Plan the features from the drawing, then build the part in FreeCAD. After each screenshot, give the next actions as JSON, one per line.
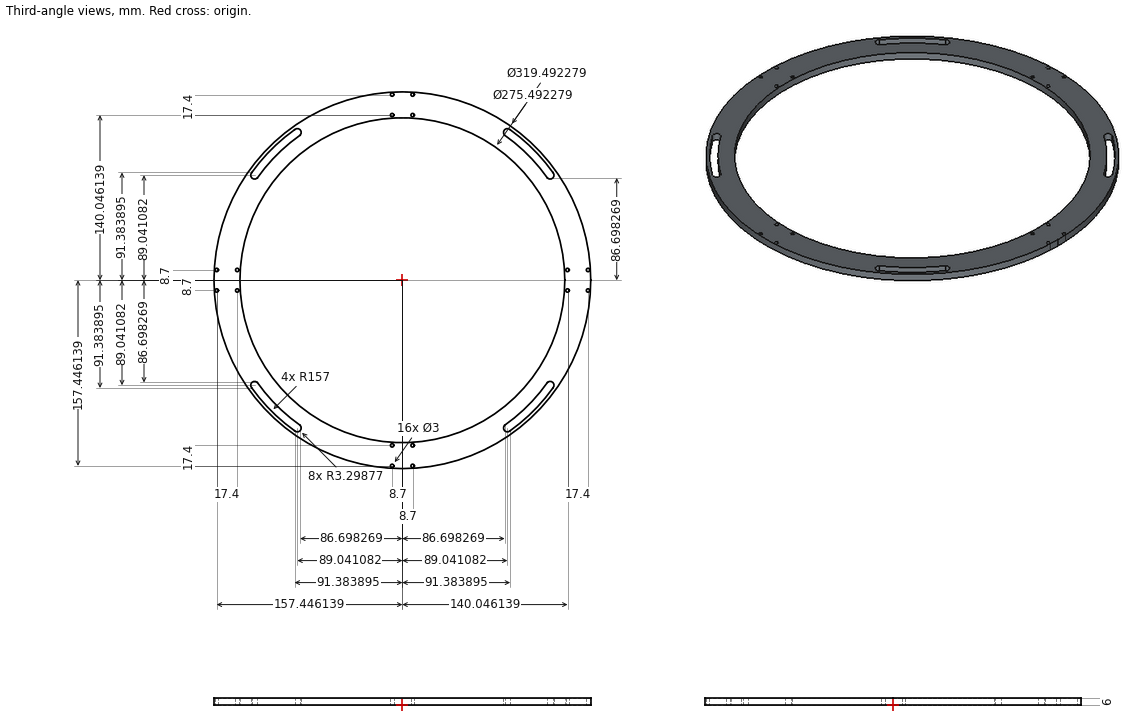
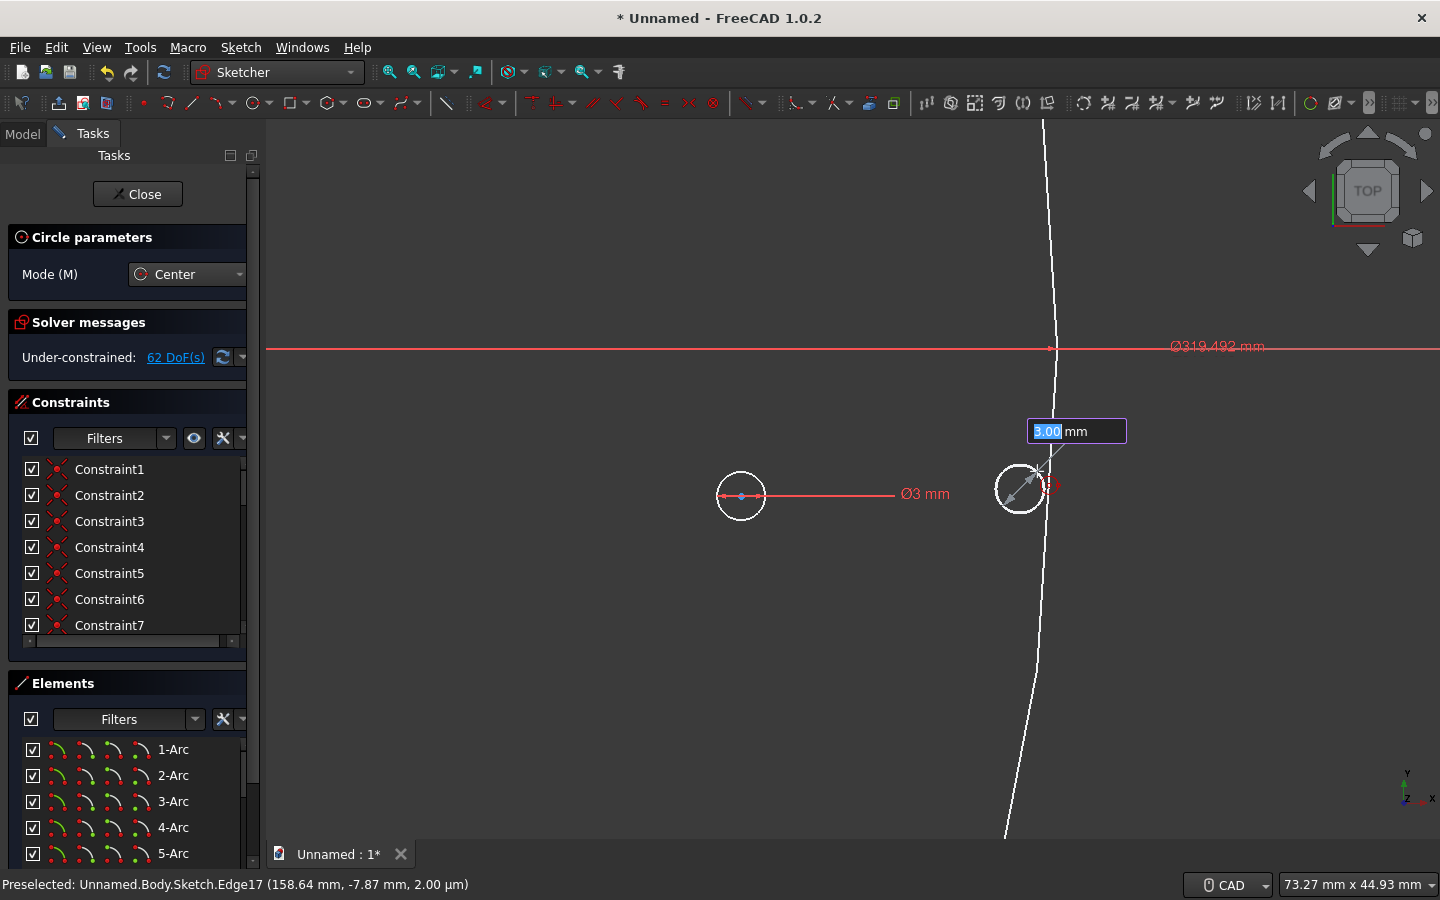
{"action": "type", "text": "3"}
{"action": "key", "text": "Return"}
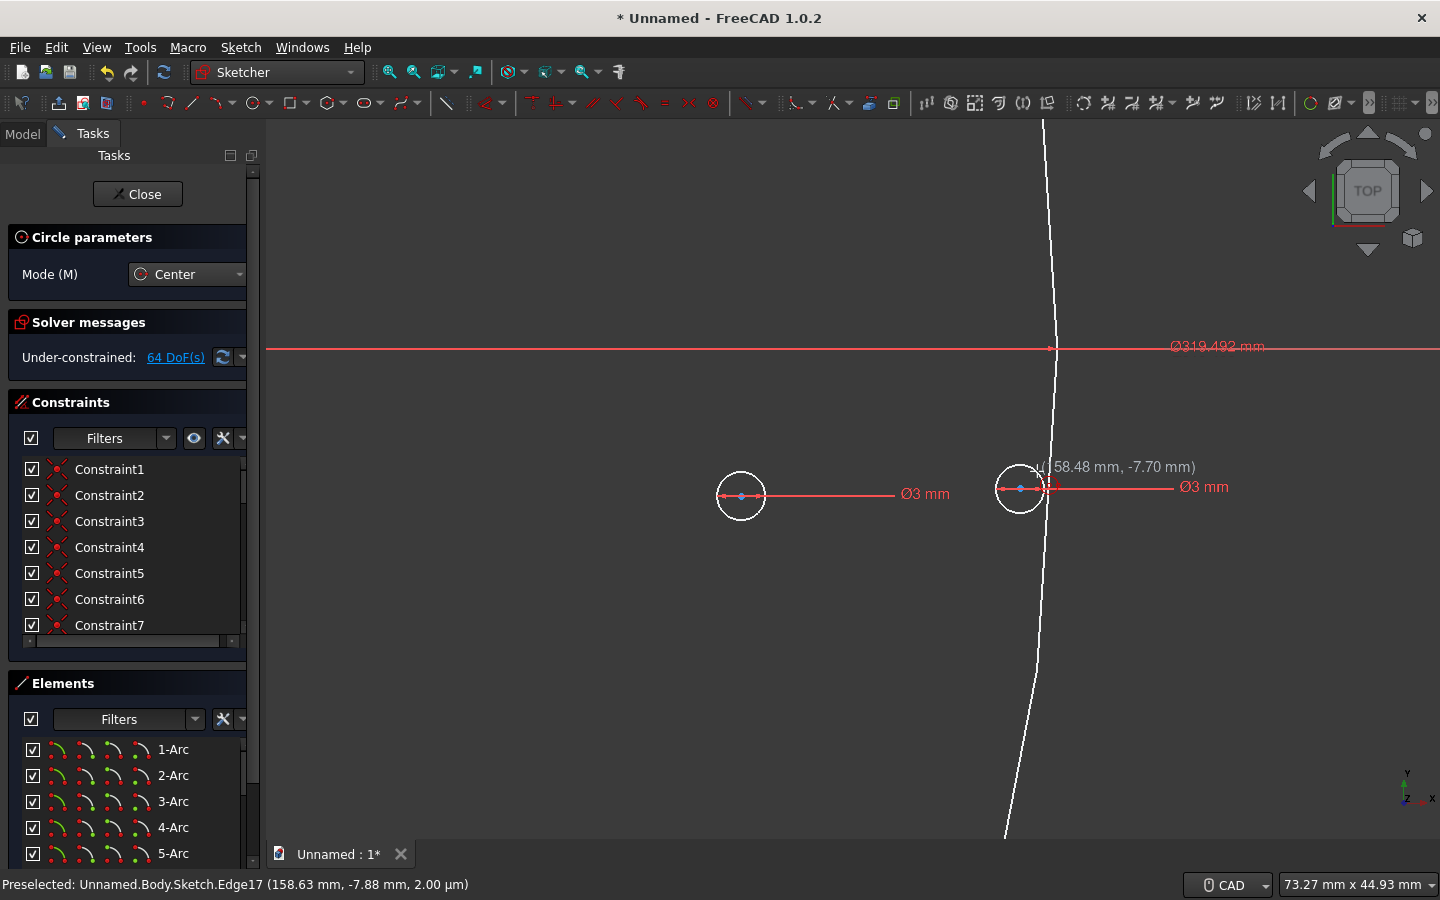
{"action": "scroll", "coordinate": [1013, 492], "scroll_direction": "down", "scroll_amount": 12}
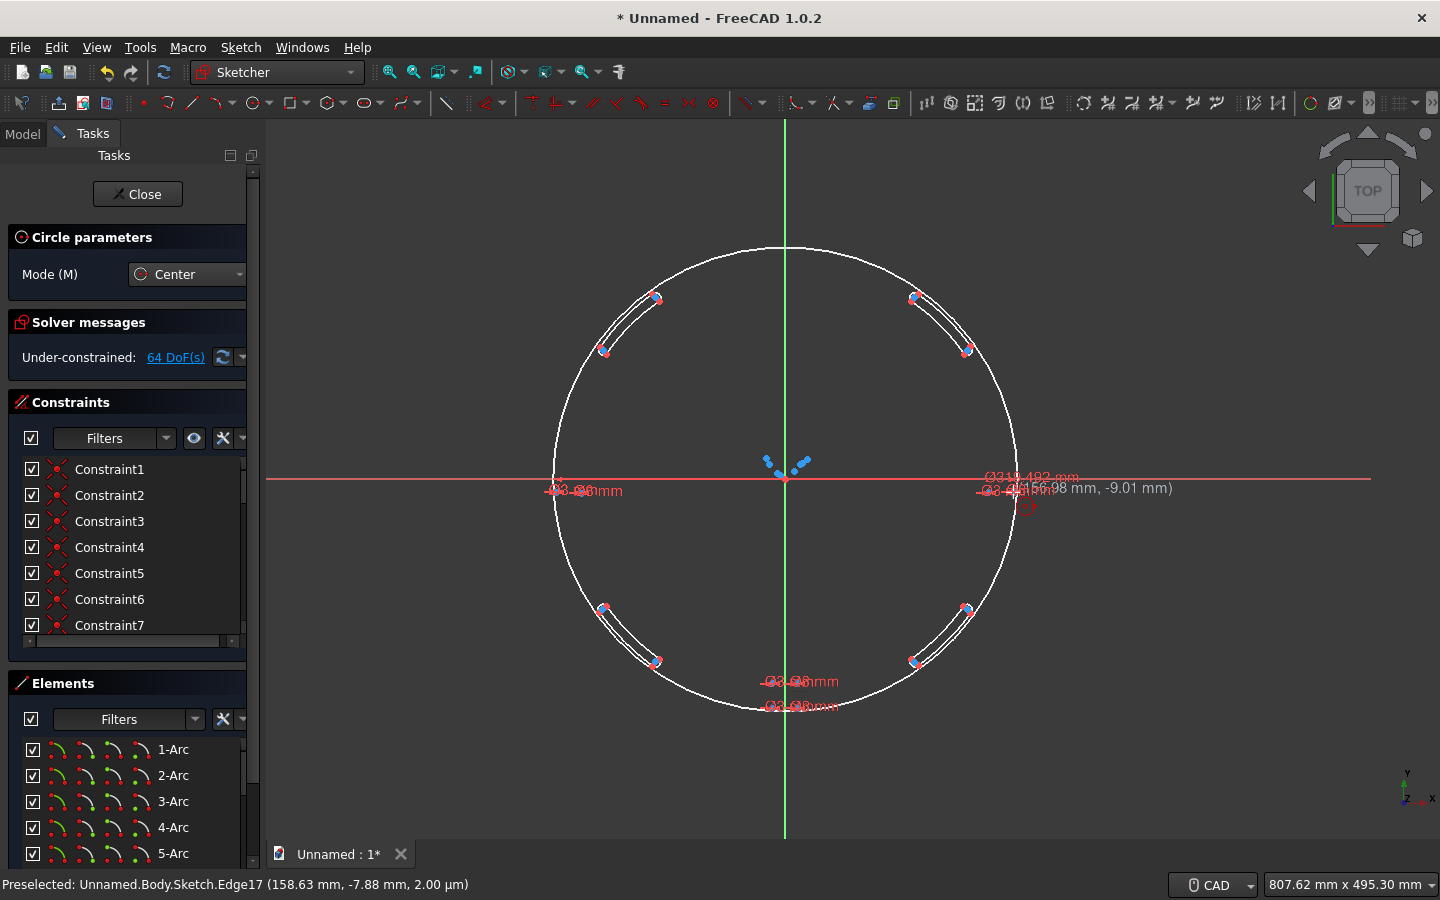
{"action": "scroll", "coordinate": [557, 467], "scroll_direction": "up", "scroll_amount": 12}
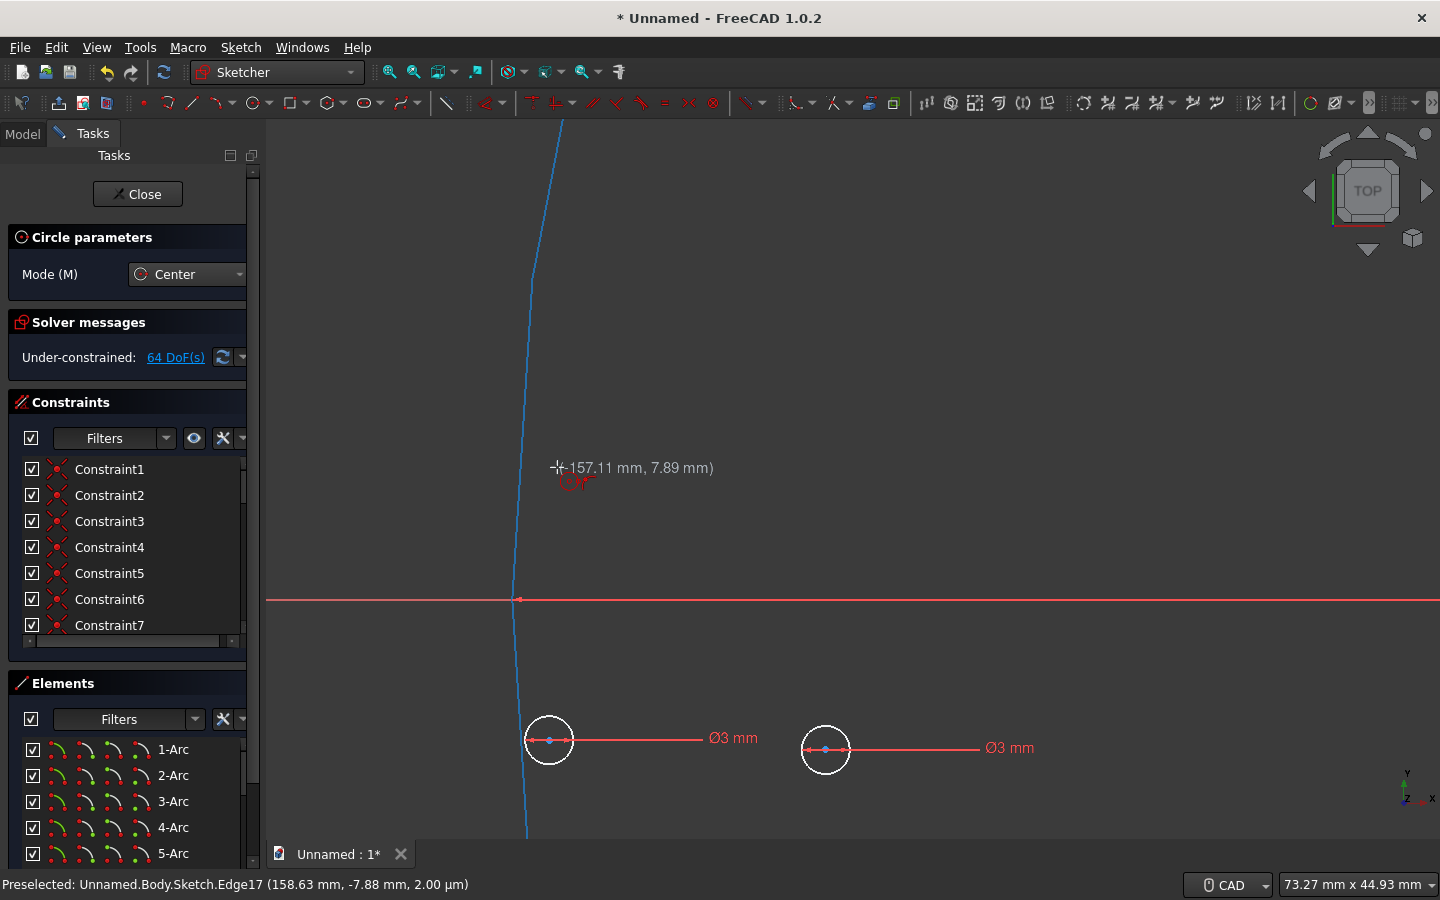
{"action": "left_click", "coordinate": [549, 460]}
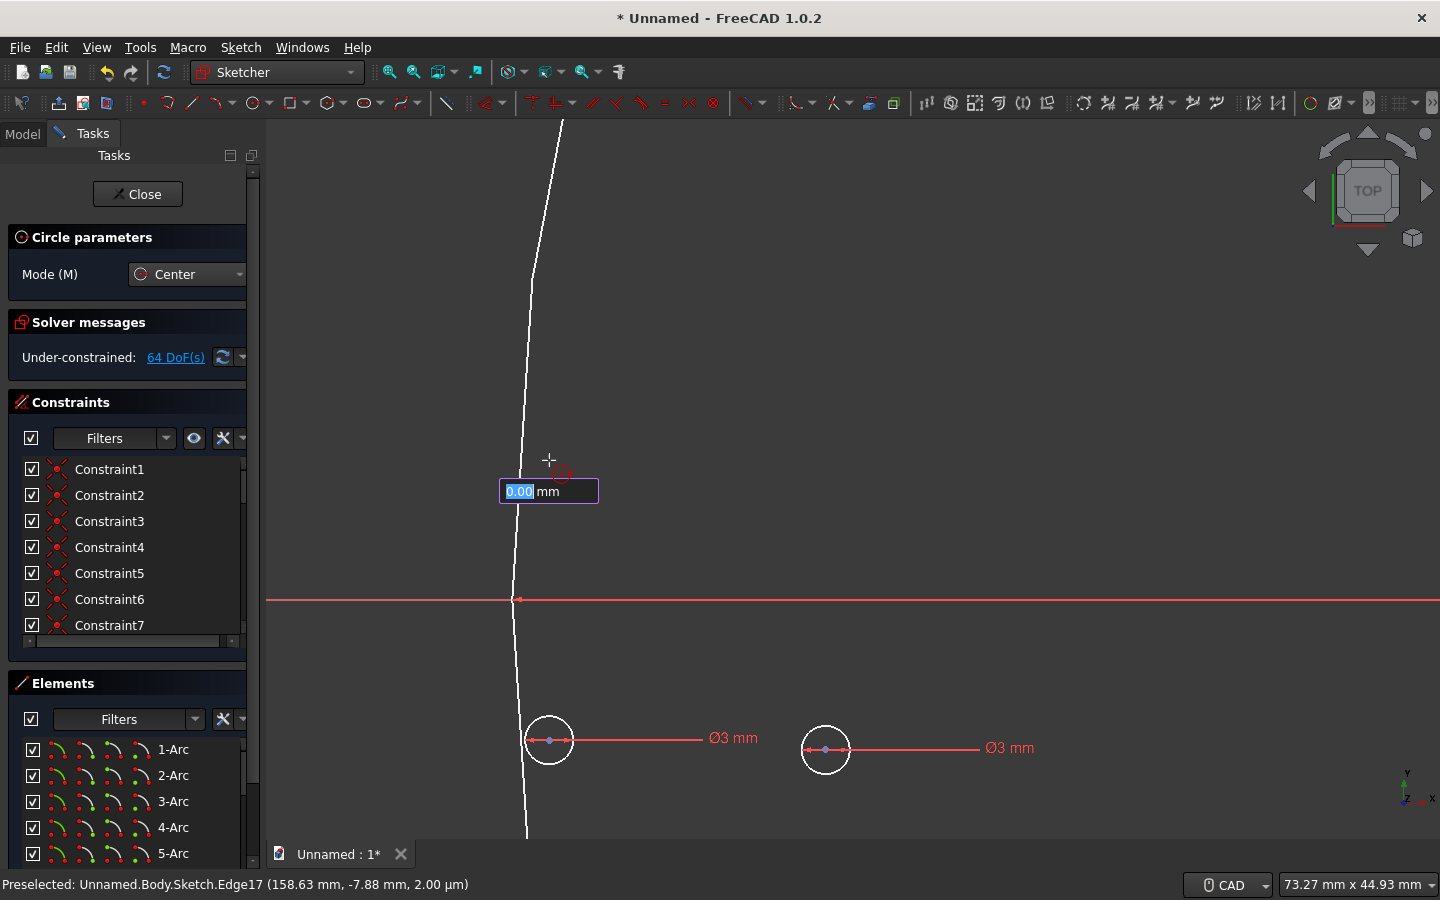
{"action": "scroll", "coordinate": [556, 467], "scroll_direction": "down", "scroll_amount": 12}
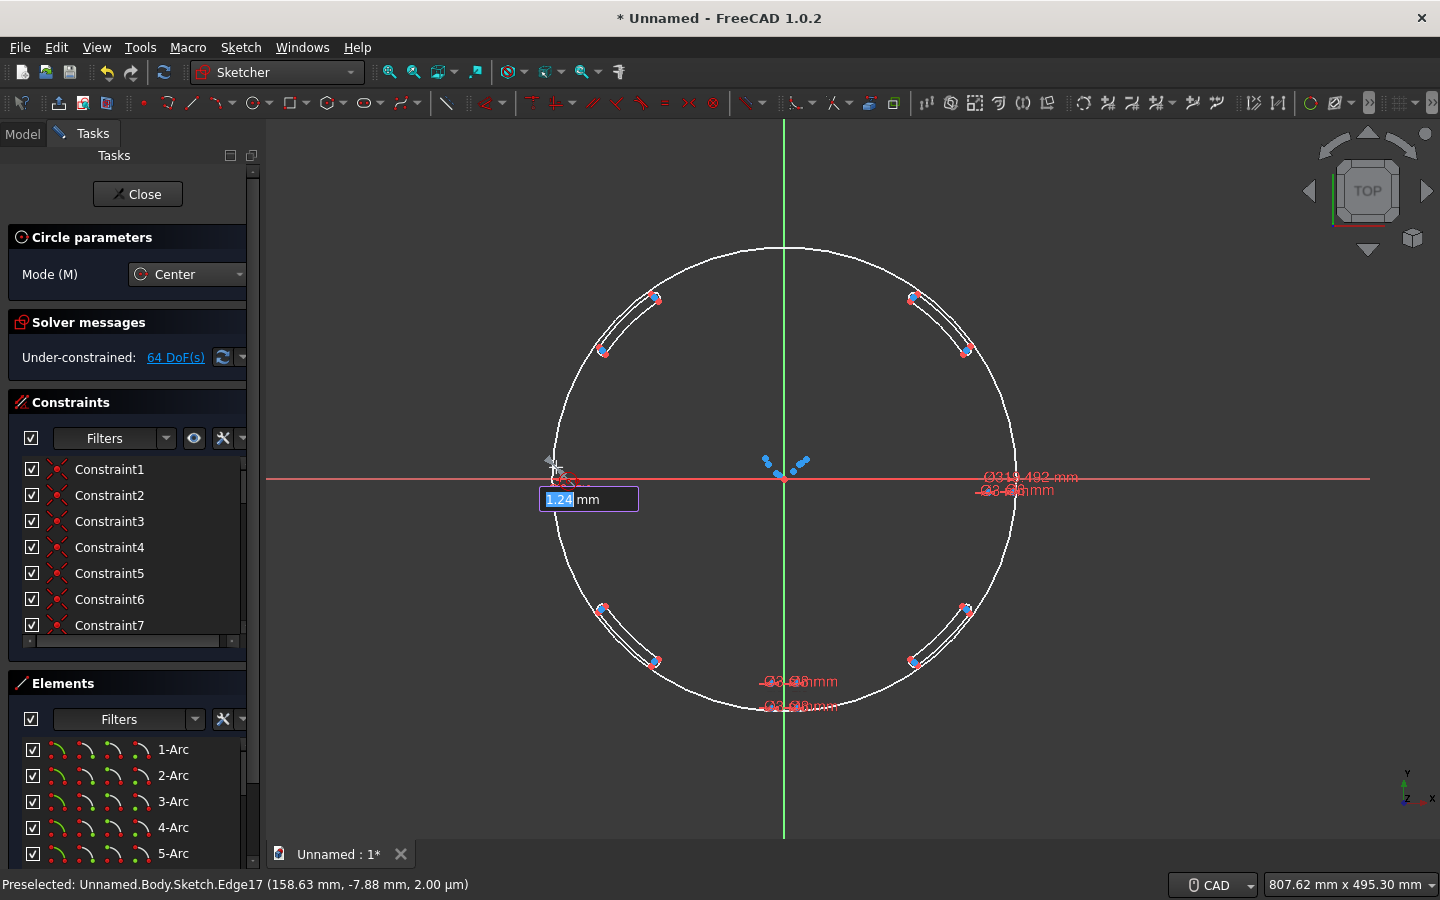
{"action": "scroll", "coordinate": [557, 465], "scroll_direction": "up", "scroll_amount": 7}
{"action": "mouse_move", "coordinate": [557, 465]}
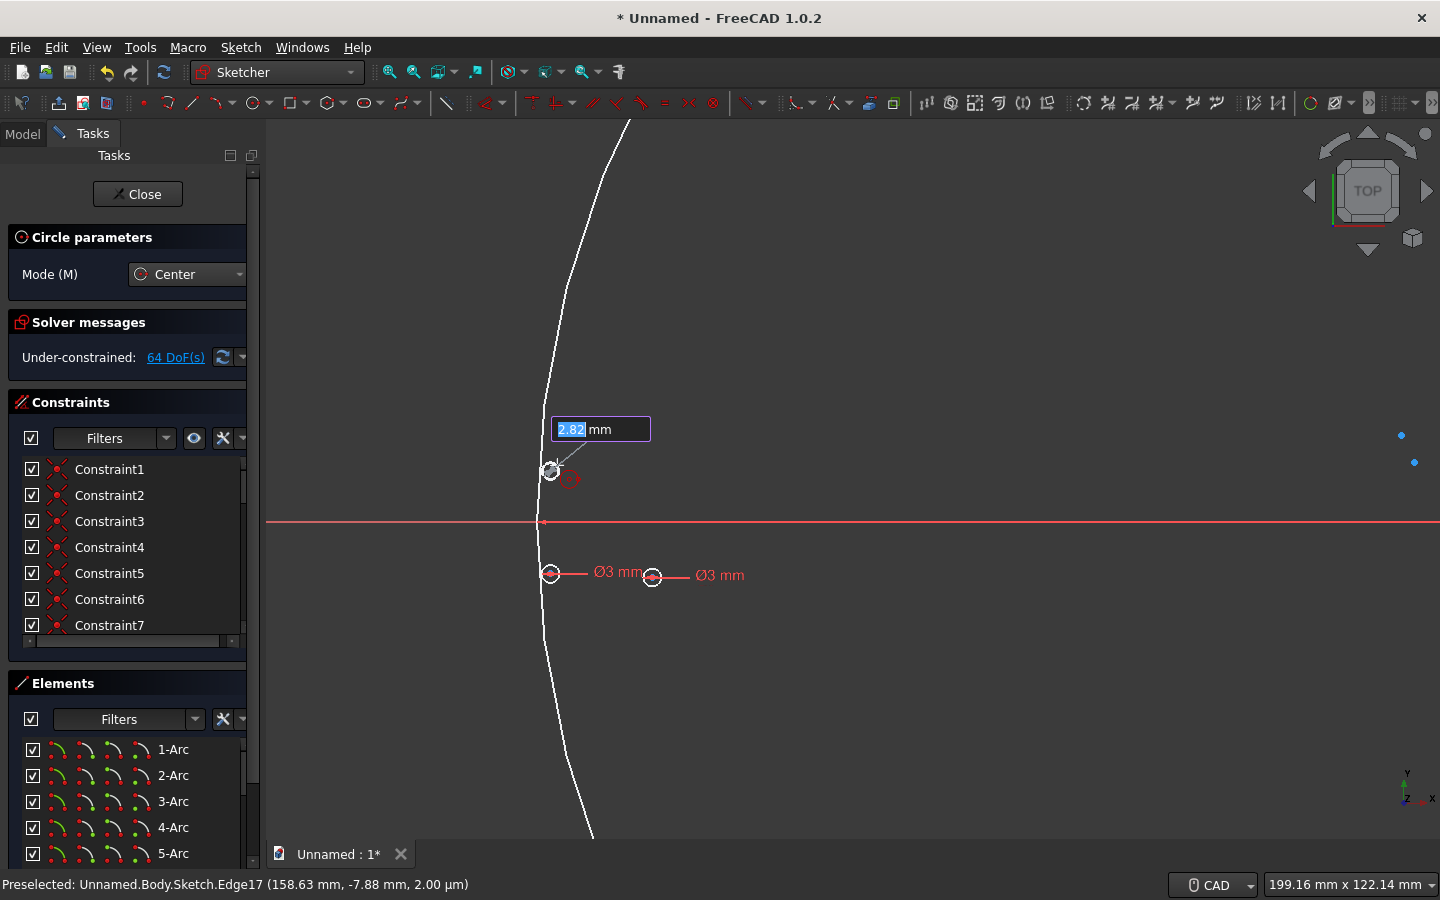
{"action": "type", "text": "3"}
{"action": "key", "text": "Return"}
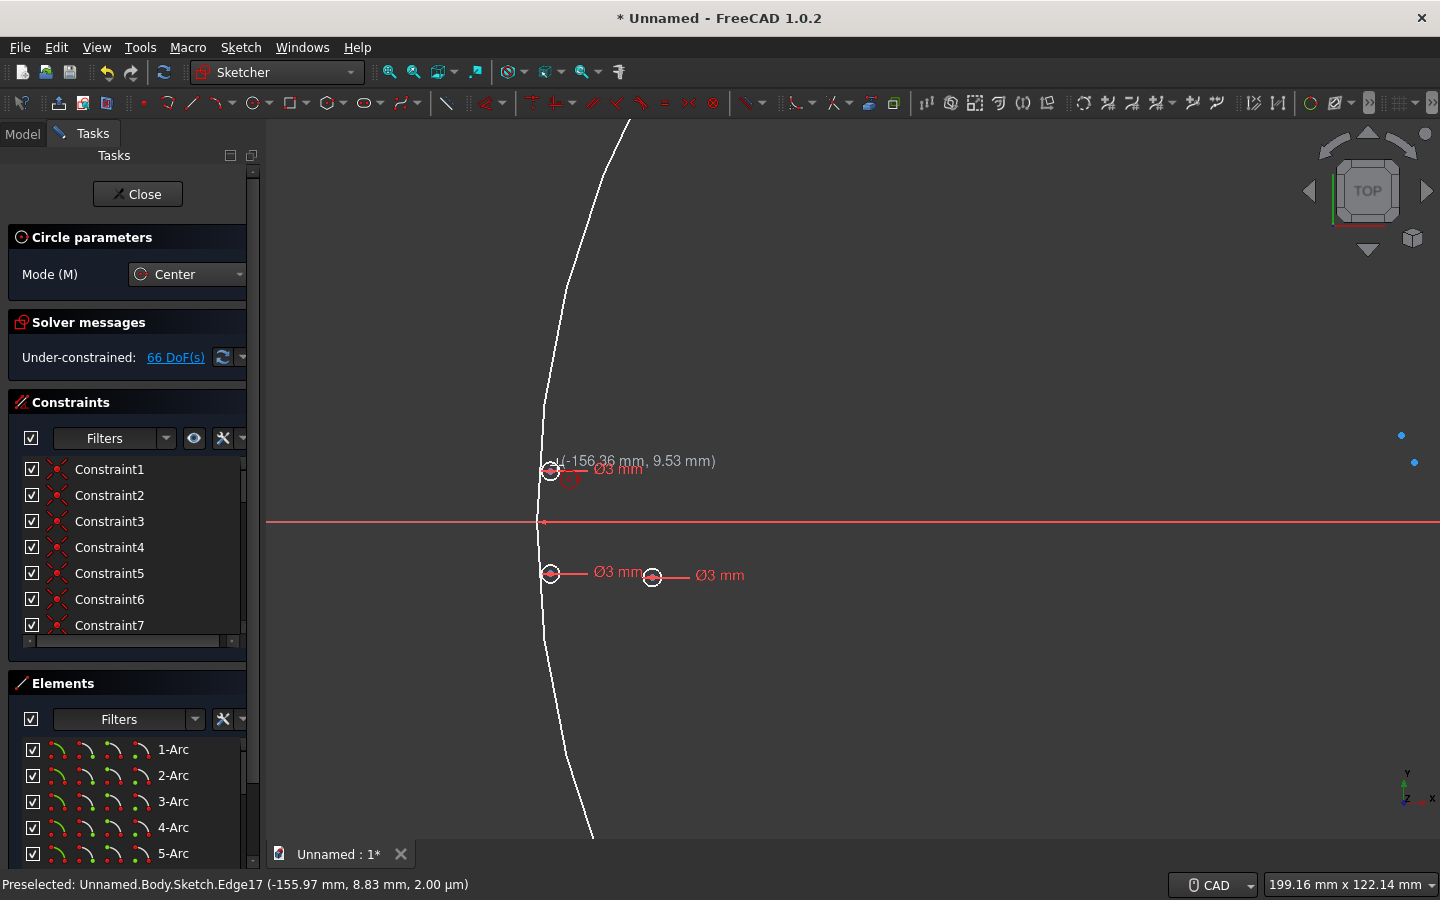
{"action": "scroll", "coordinate": [653, 471], "scroll_direction": "up", "scroll_amount": 5}